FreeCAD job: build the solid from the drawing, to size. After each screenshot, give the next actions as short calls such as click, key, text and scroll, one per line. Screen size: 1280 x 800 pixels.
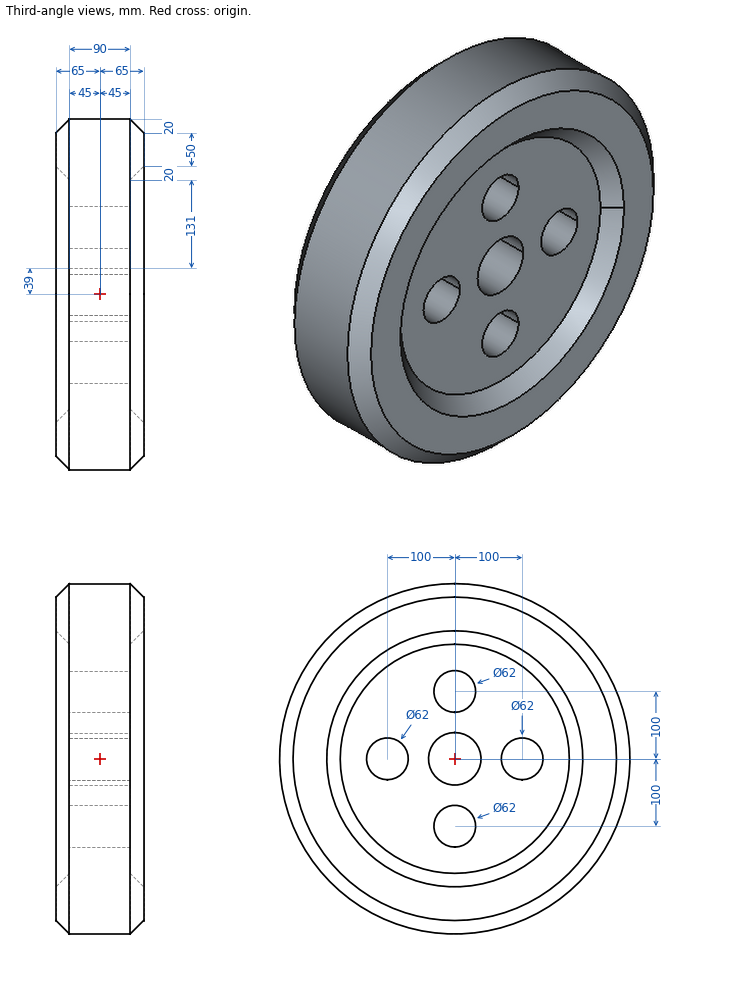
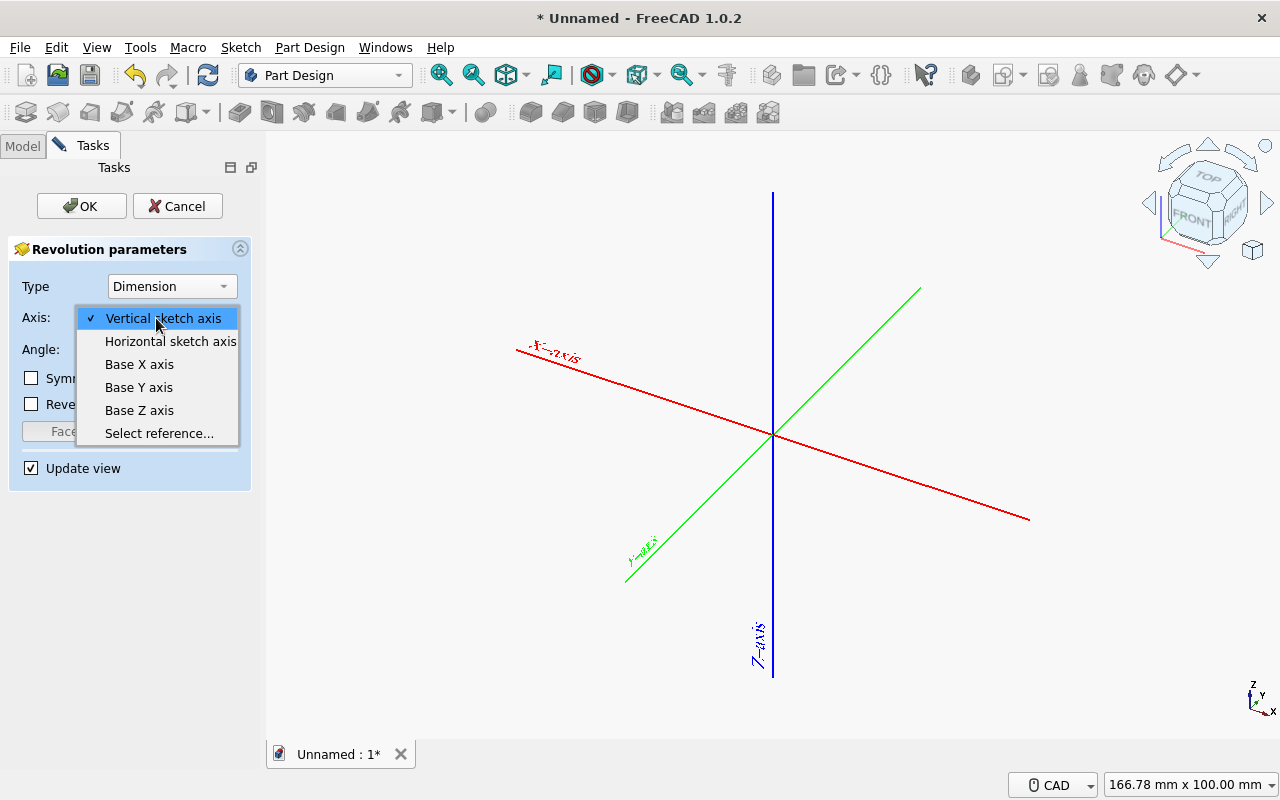
click(156, 342)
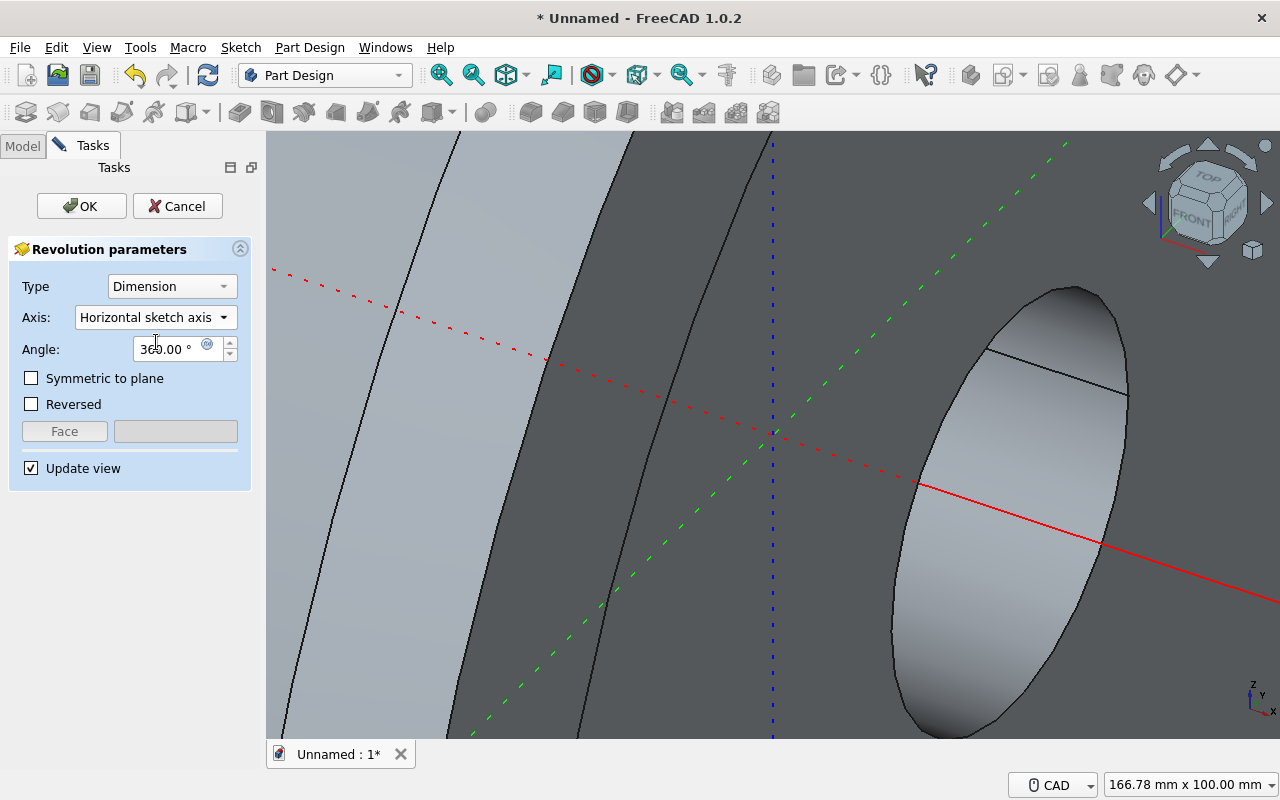
click(82, 206)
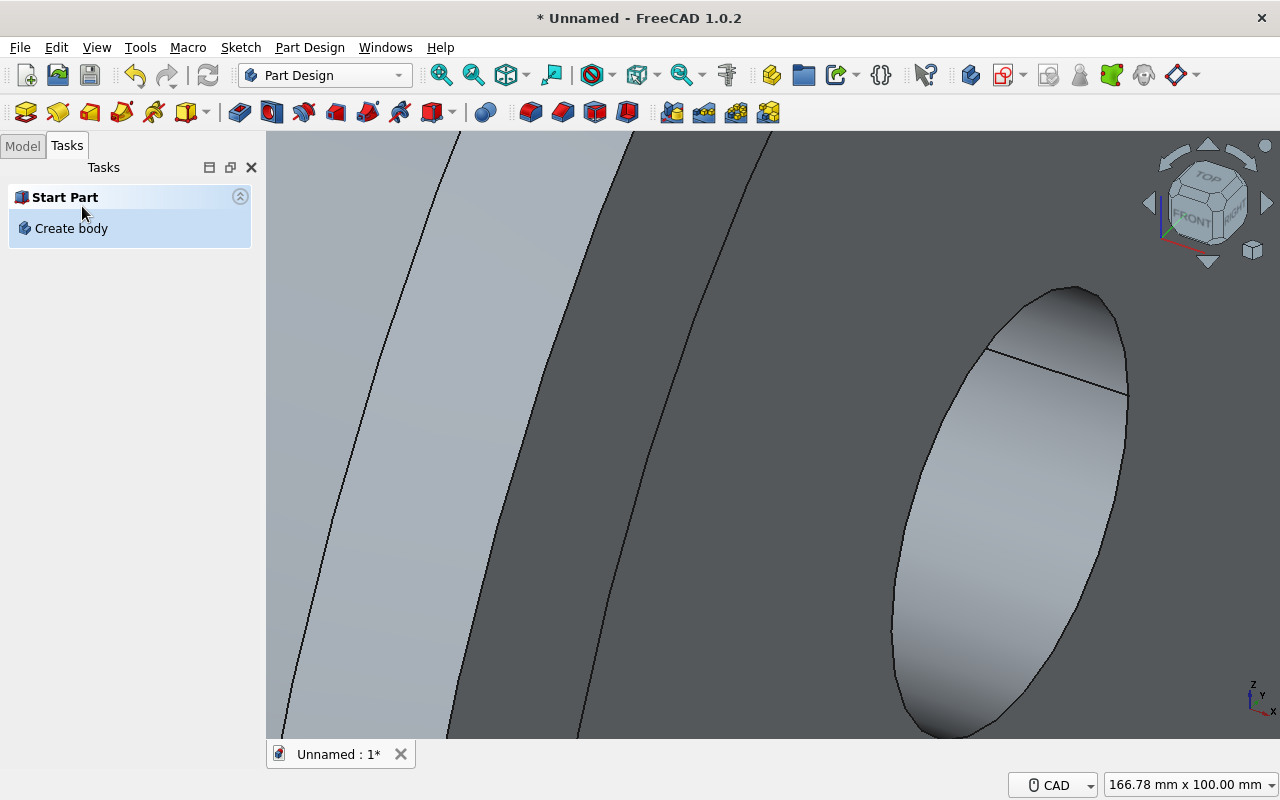
key(v)
key(f)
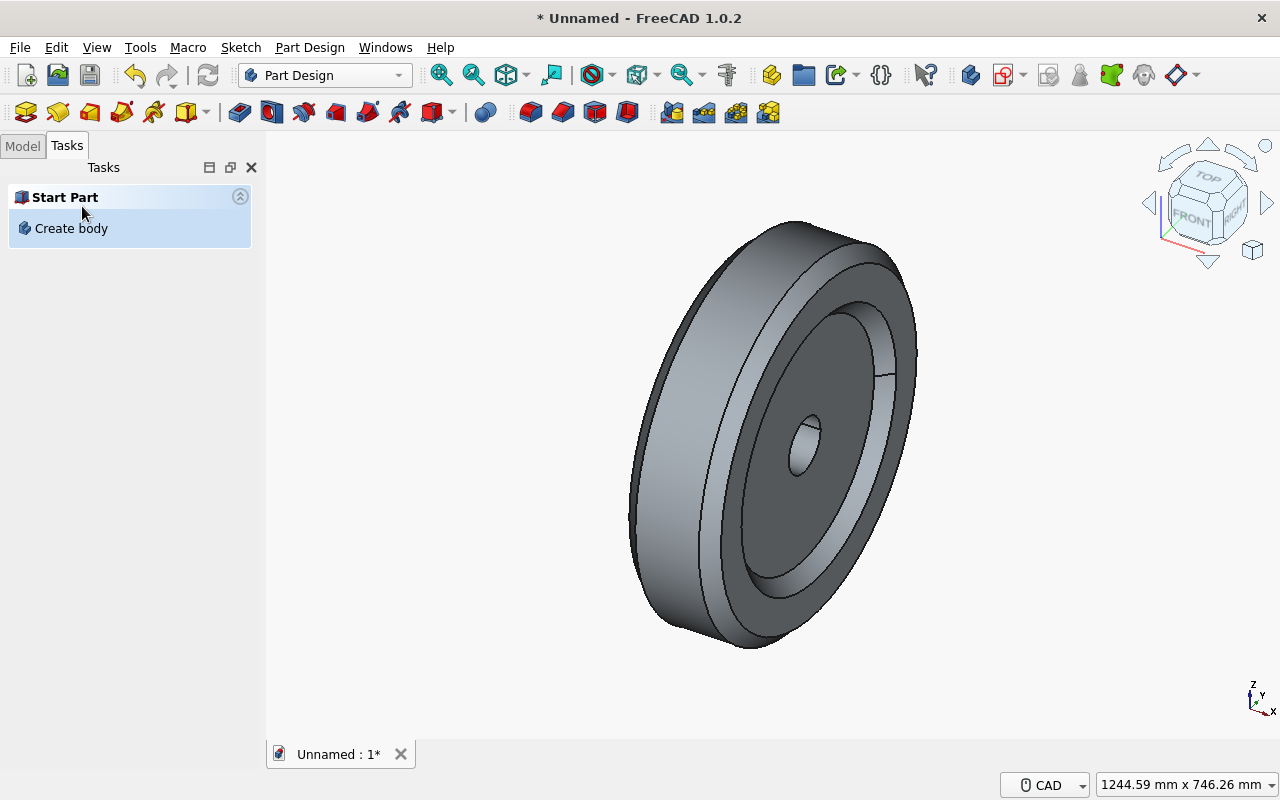
click(825, 490)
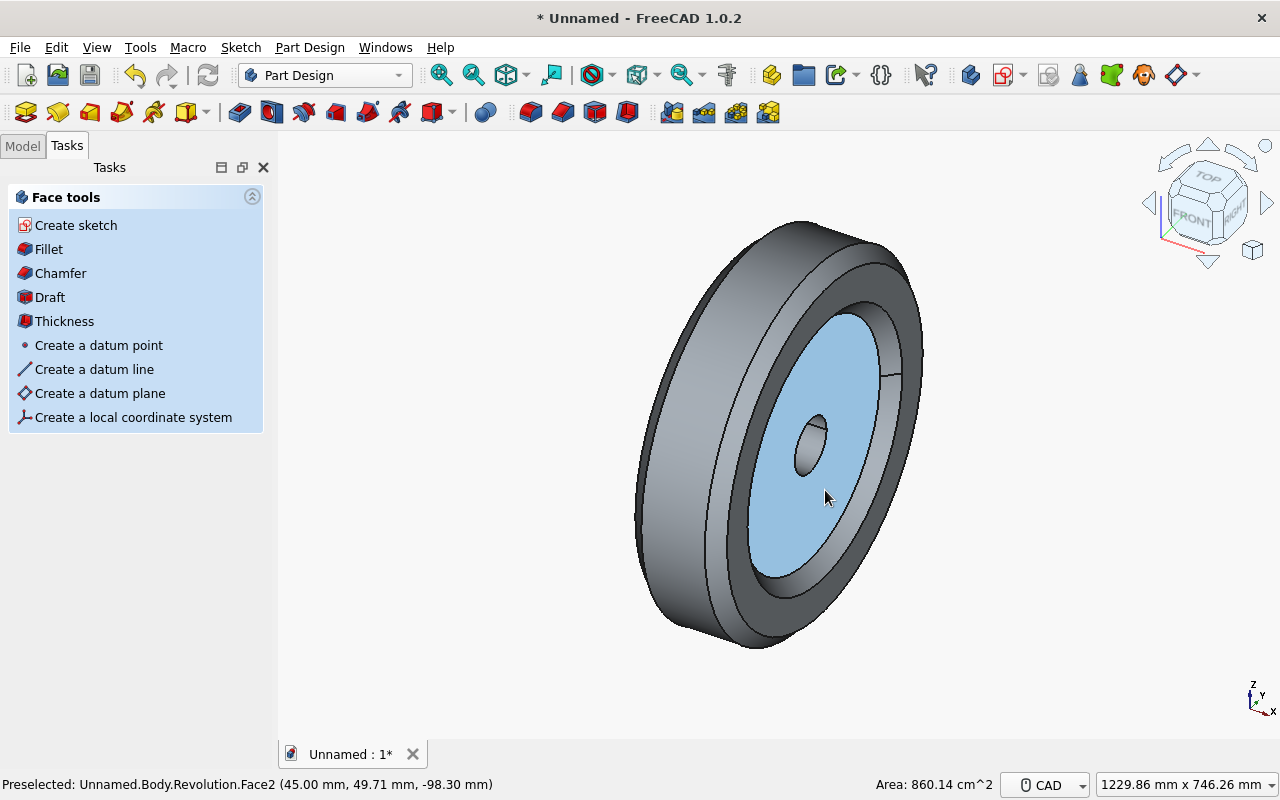
click(1004, 76)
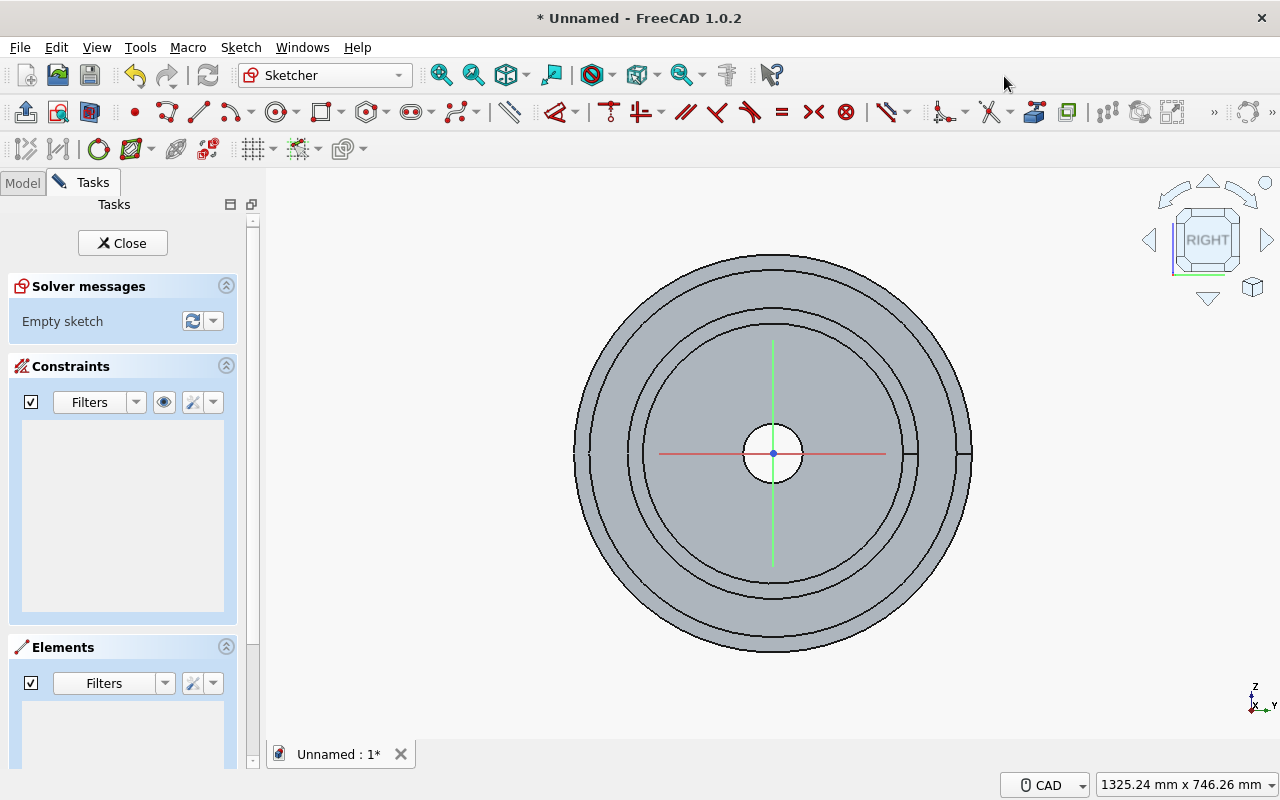
scroll(847, 454, up, 9)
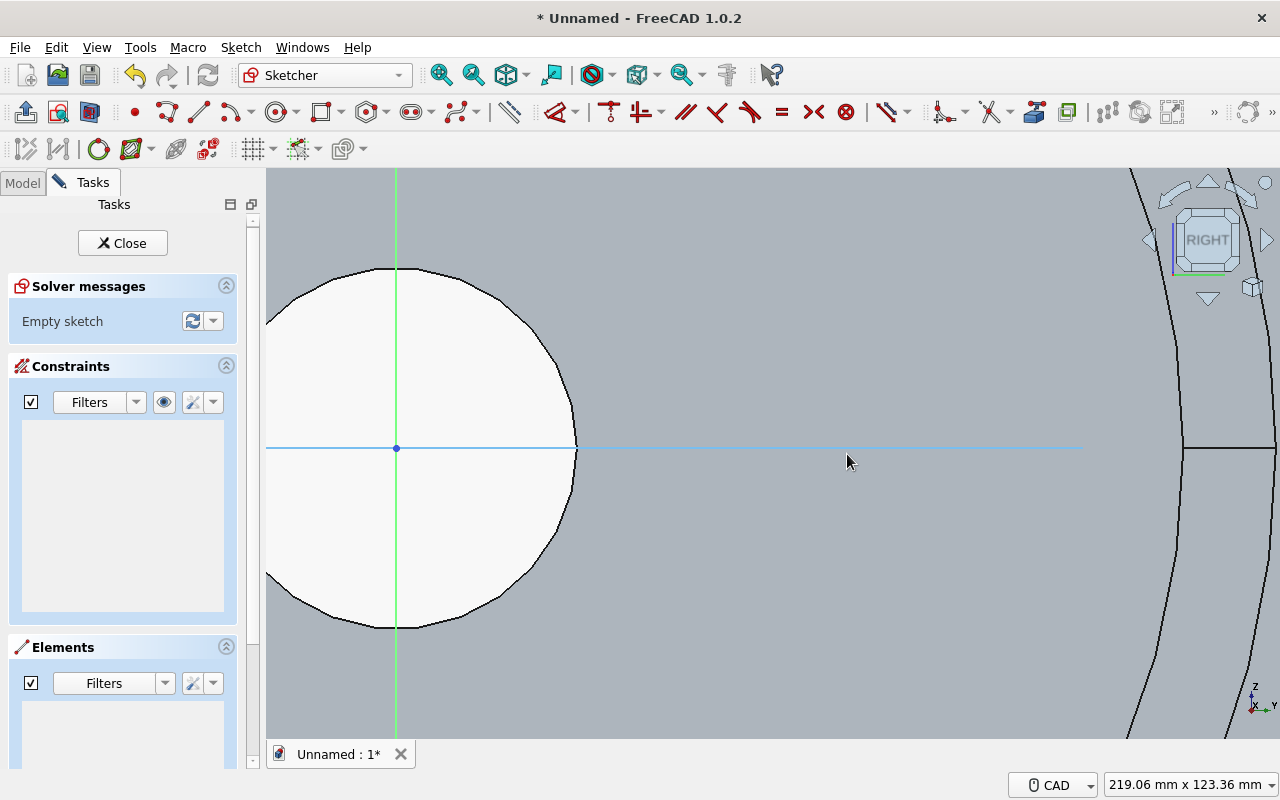
key(g)
key(c)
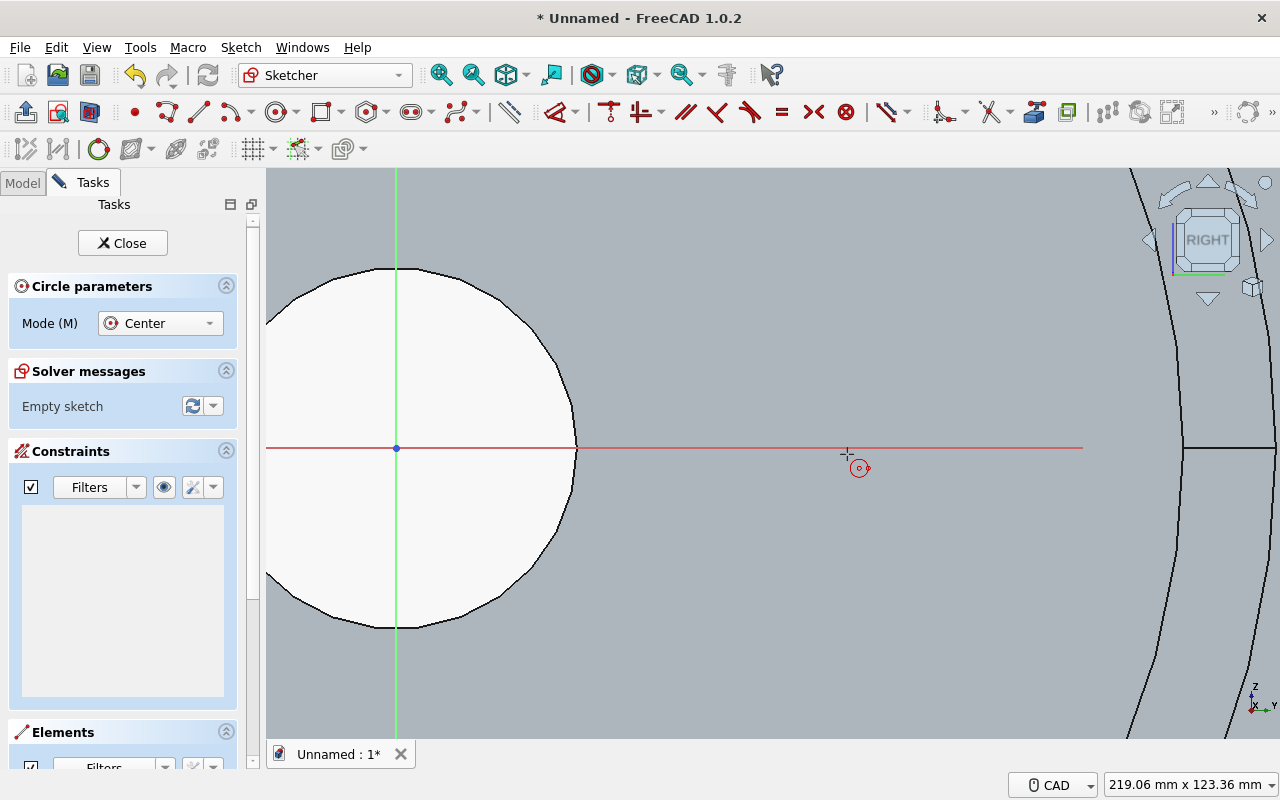
click(859, 448)
click(961, 347)
key(Escape)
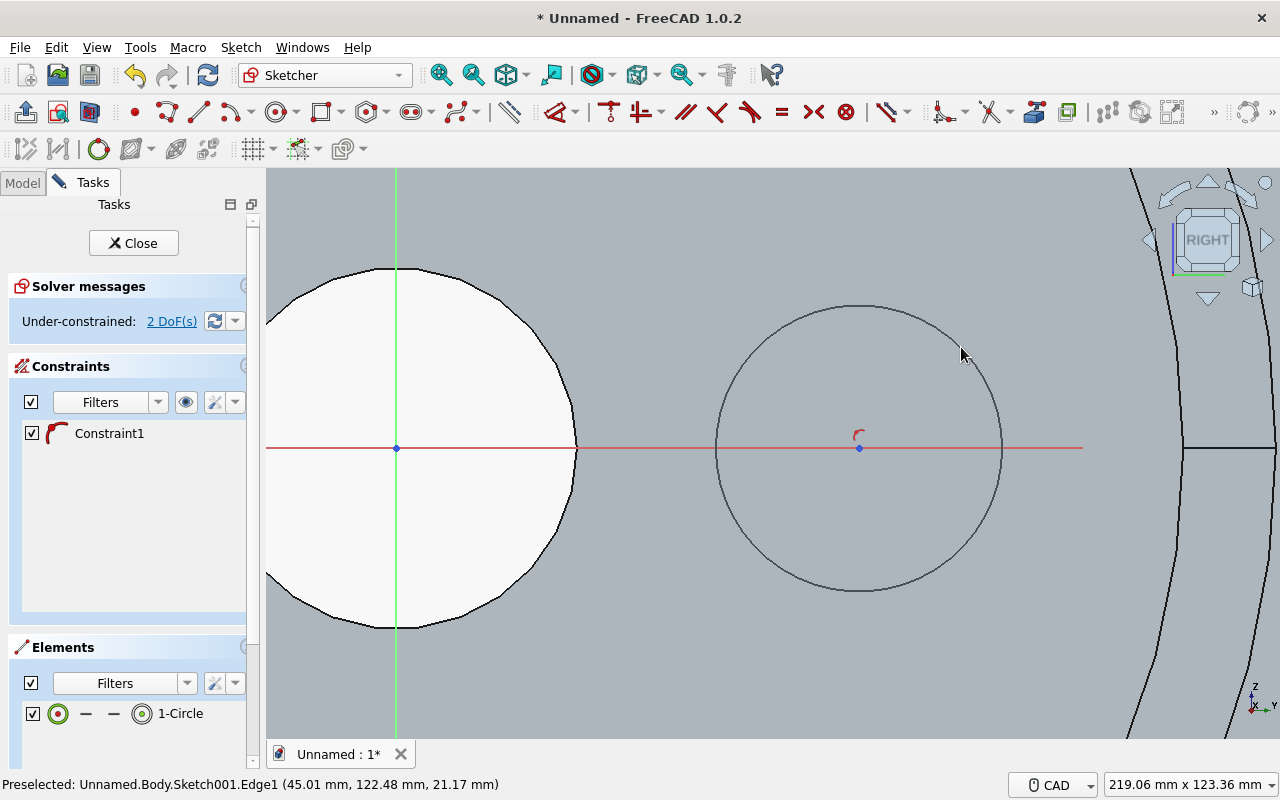
key(d)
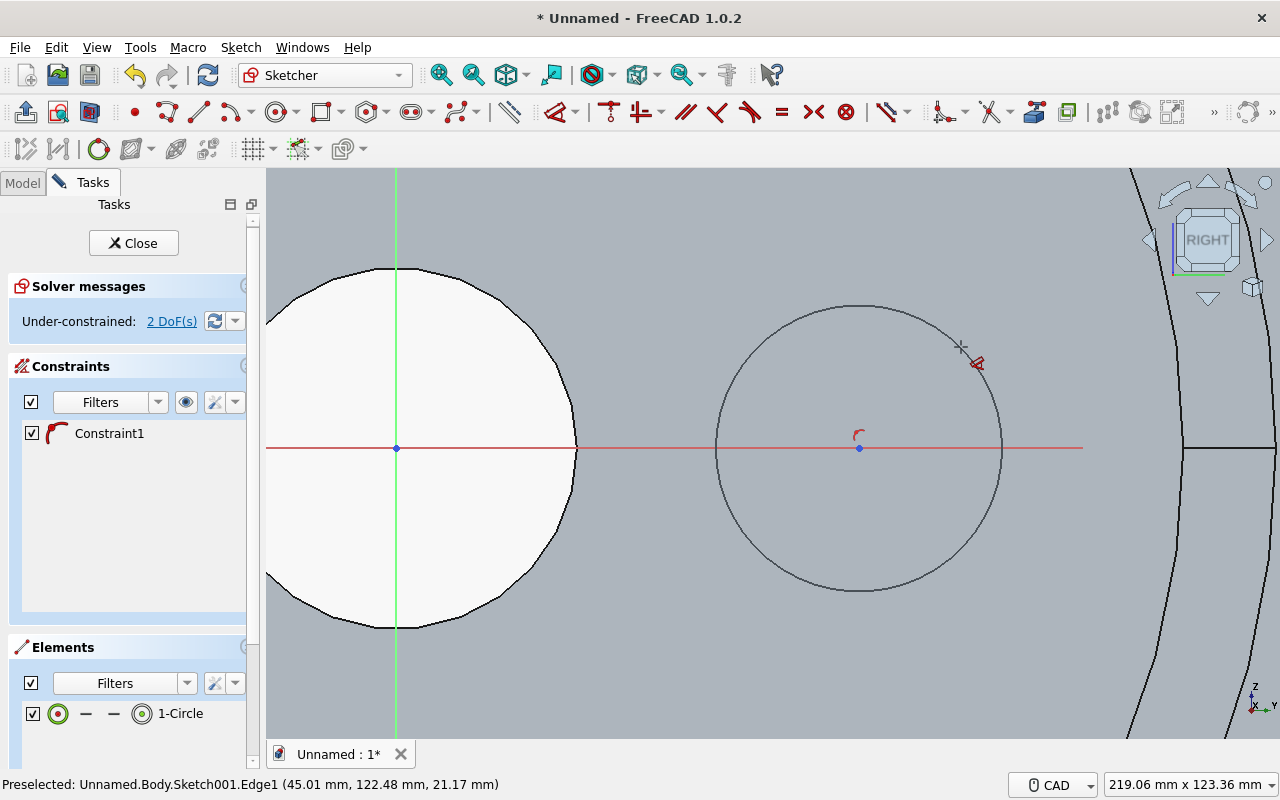
click(960, 347)
click(983, 324)